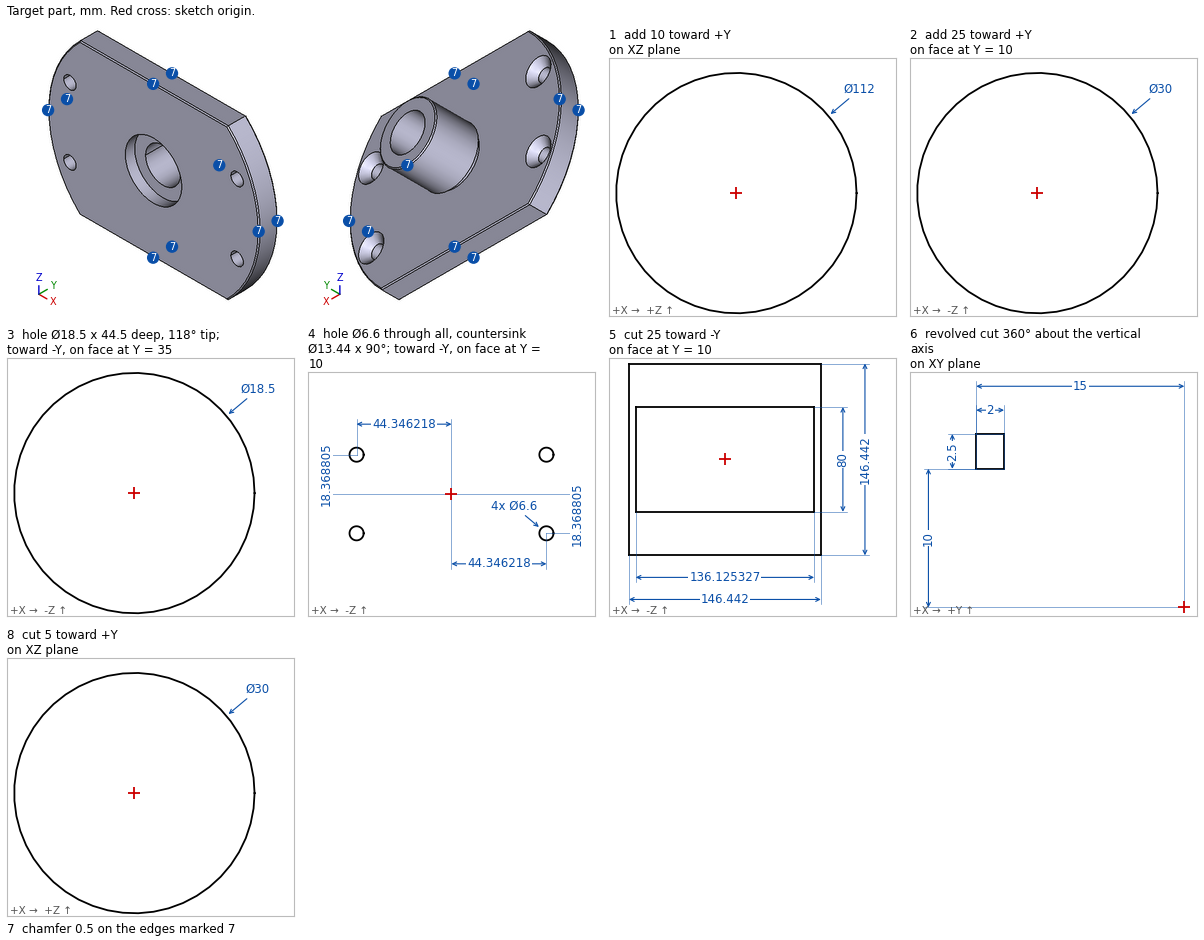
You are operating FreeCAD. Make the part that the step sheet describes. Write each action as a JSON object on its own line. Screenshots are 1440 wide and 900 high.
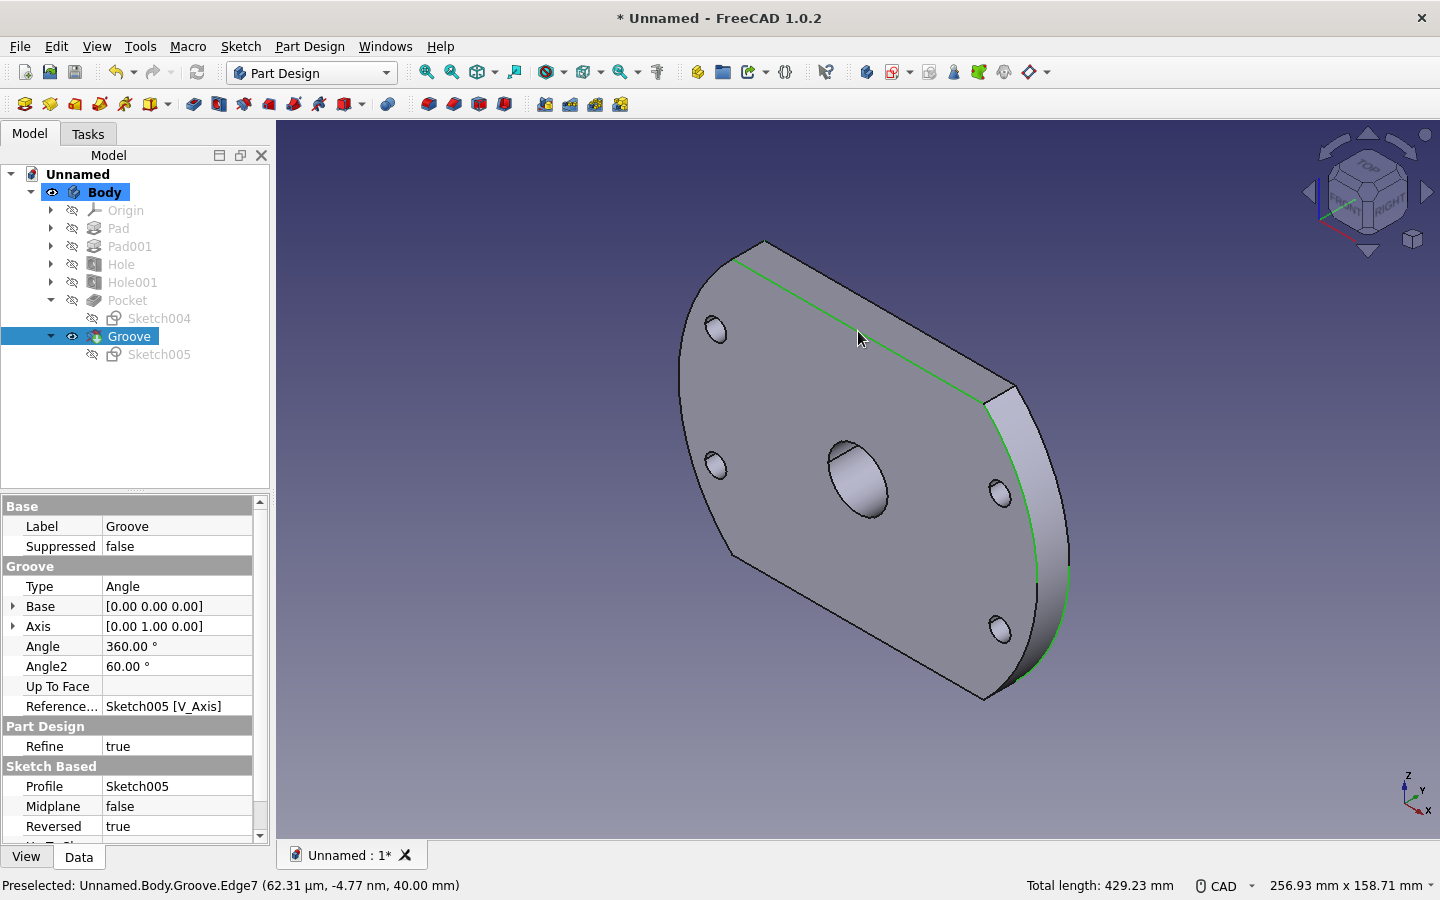
{"action": "key", "text": "2"}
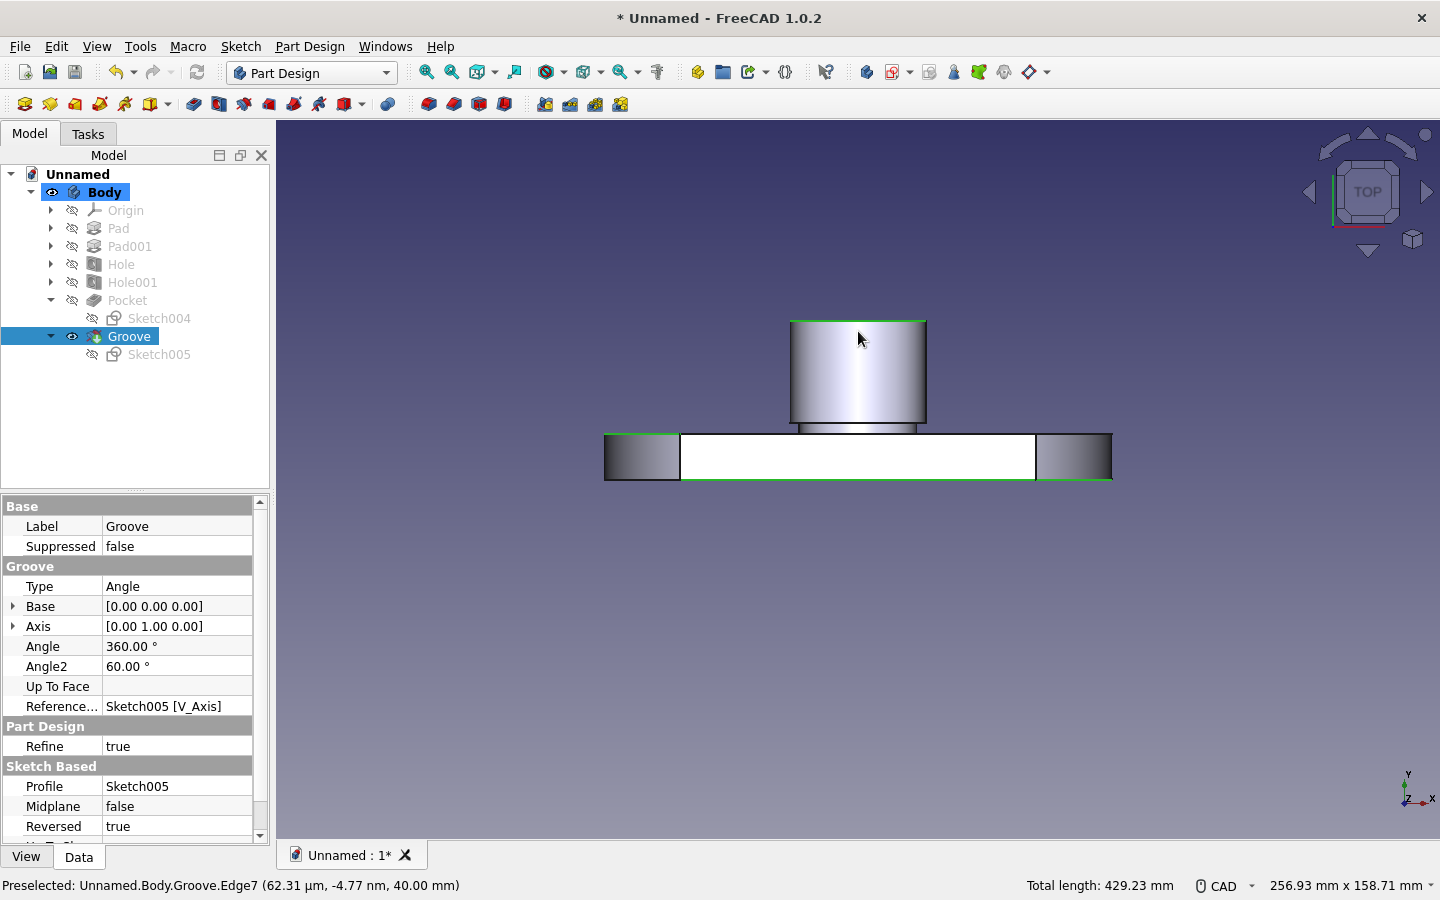
{"action": "left_click", "coordinate": [427, 72]}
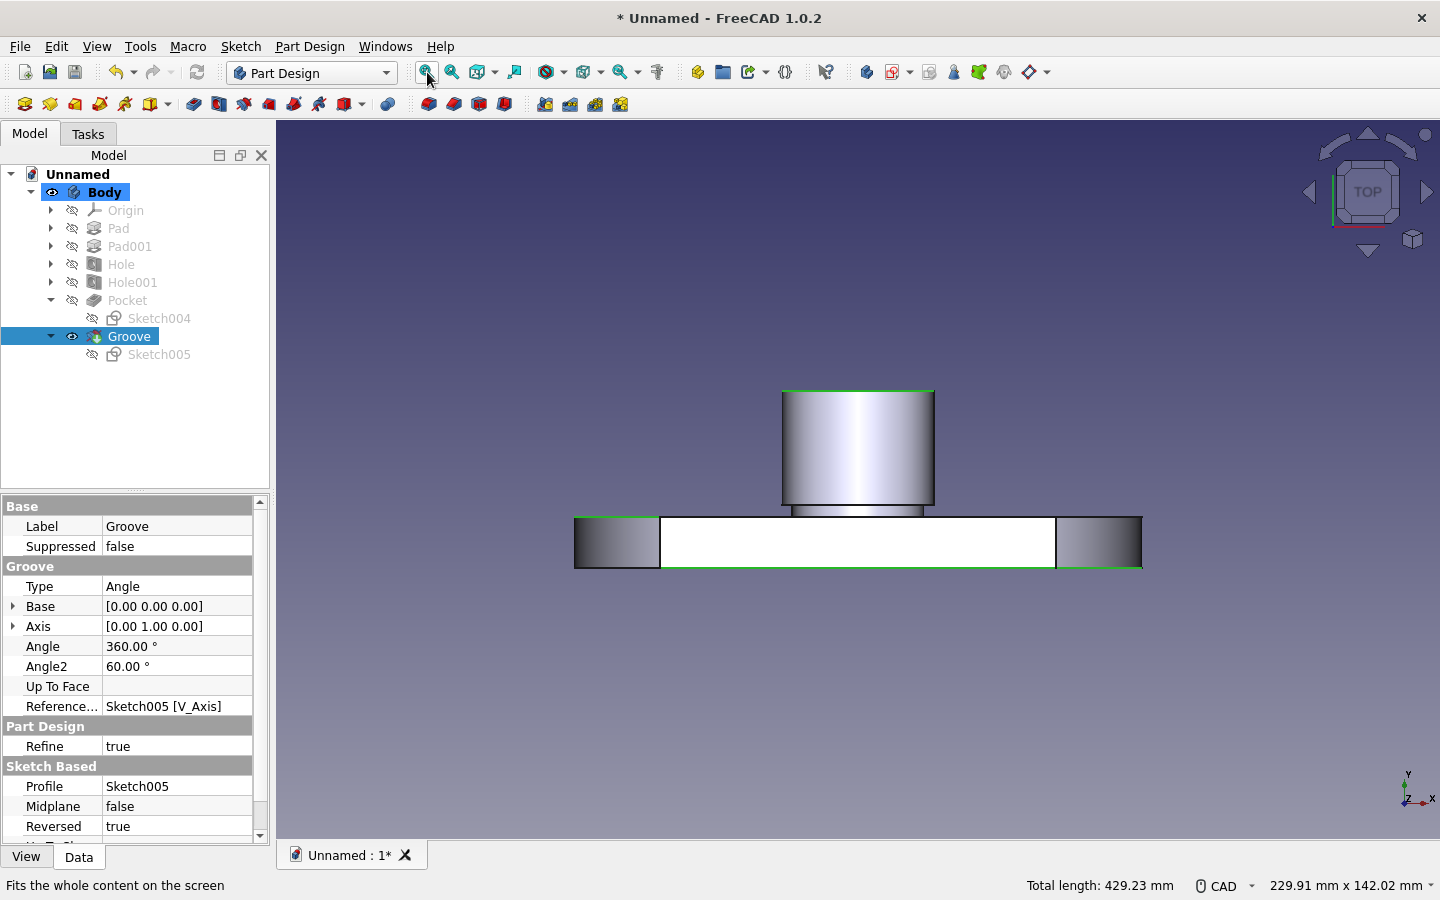
{"action": "left_click", "coordinate": [858, 516], "text": "ctrl"}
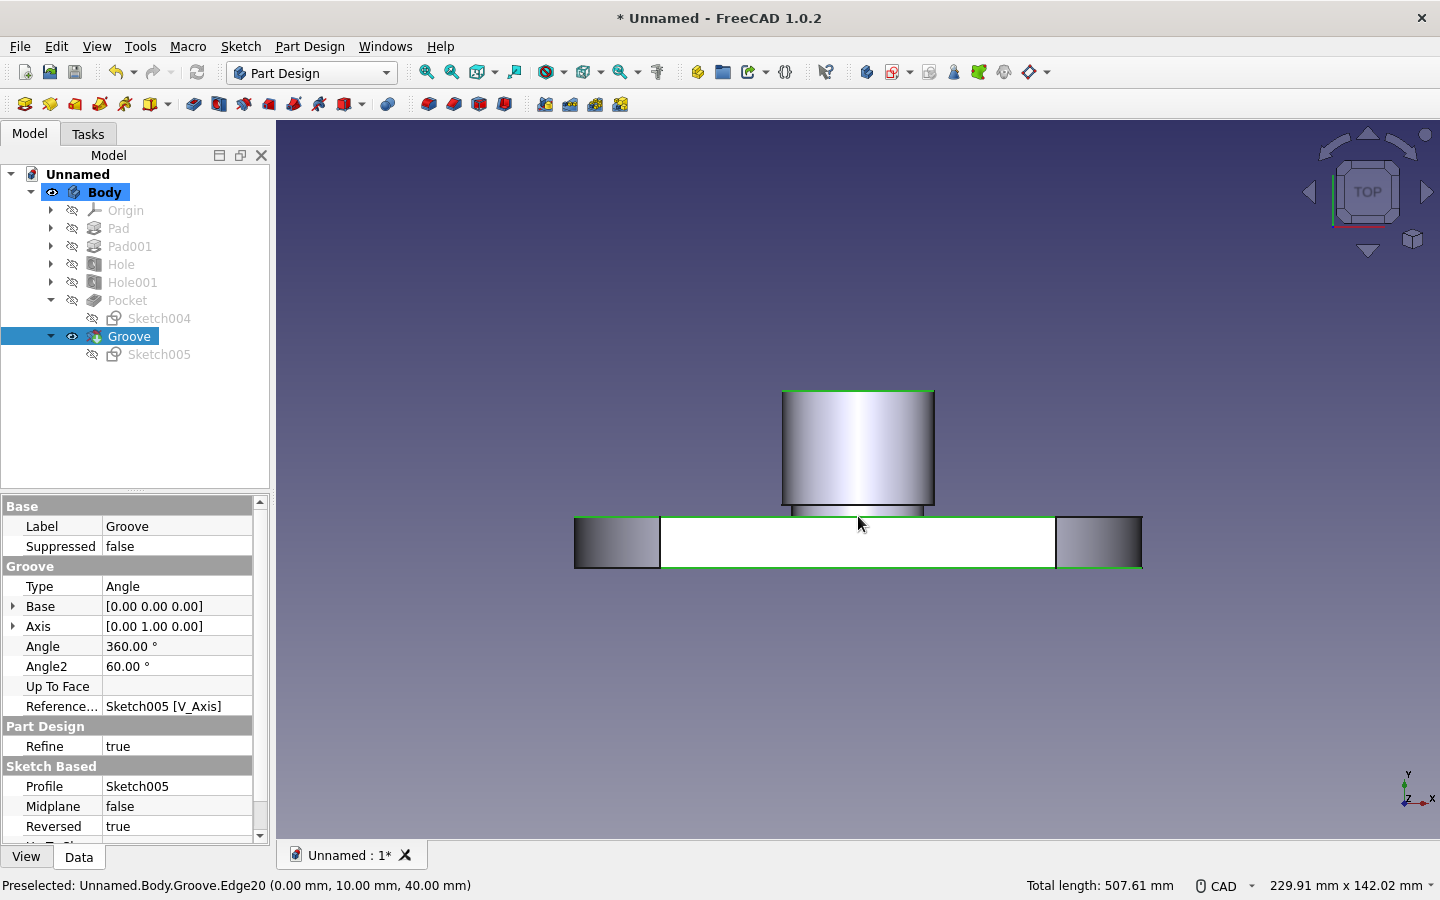
{"action": "key", "text": "1"}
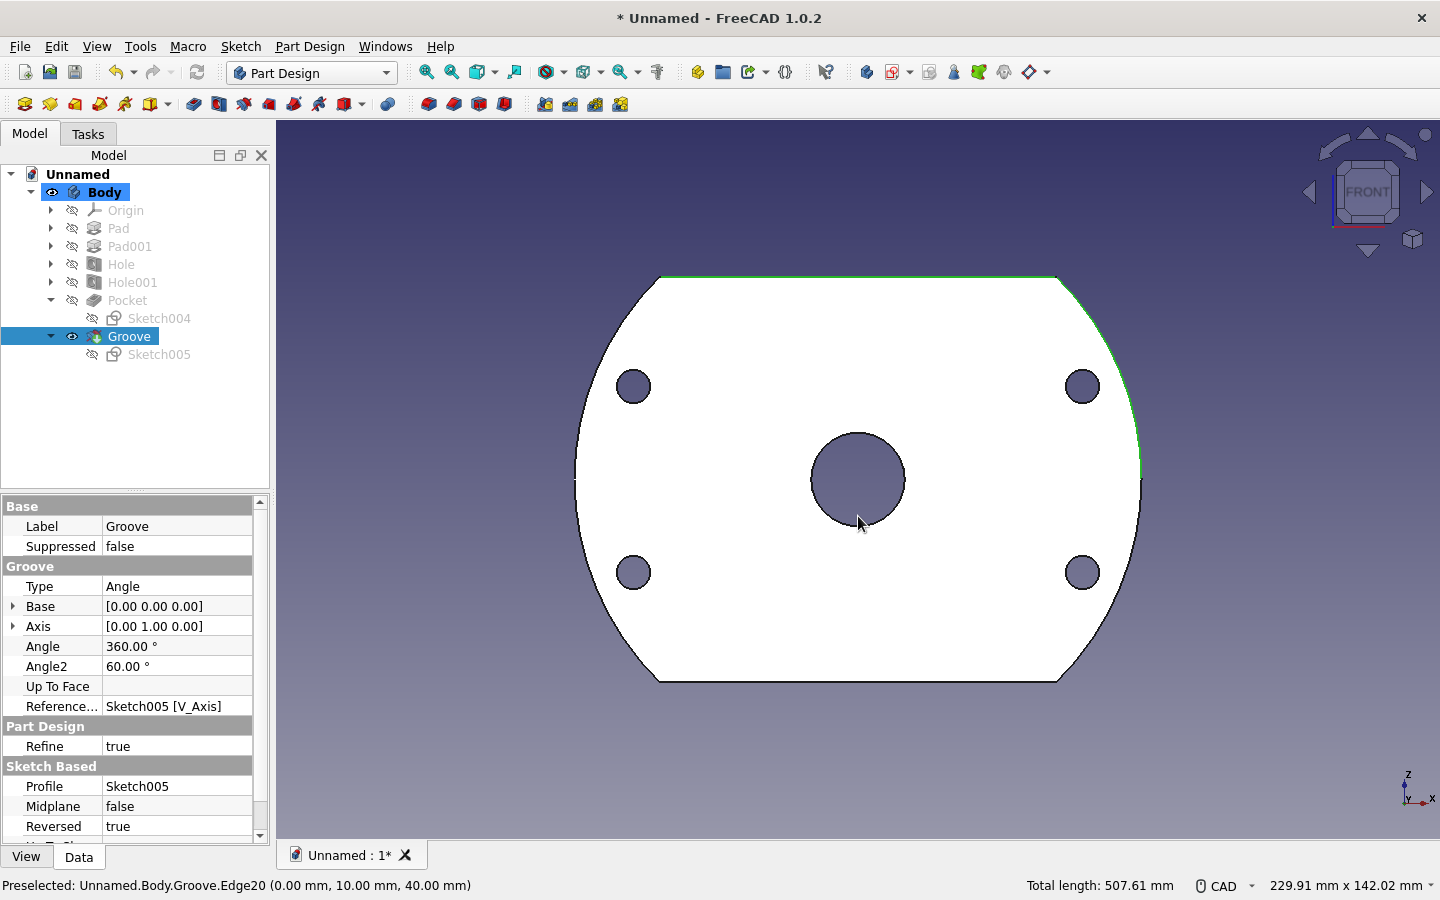
{"action": "left_click", "coordinate": [574, 478], "text": "ctrl"}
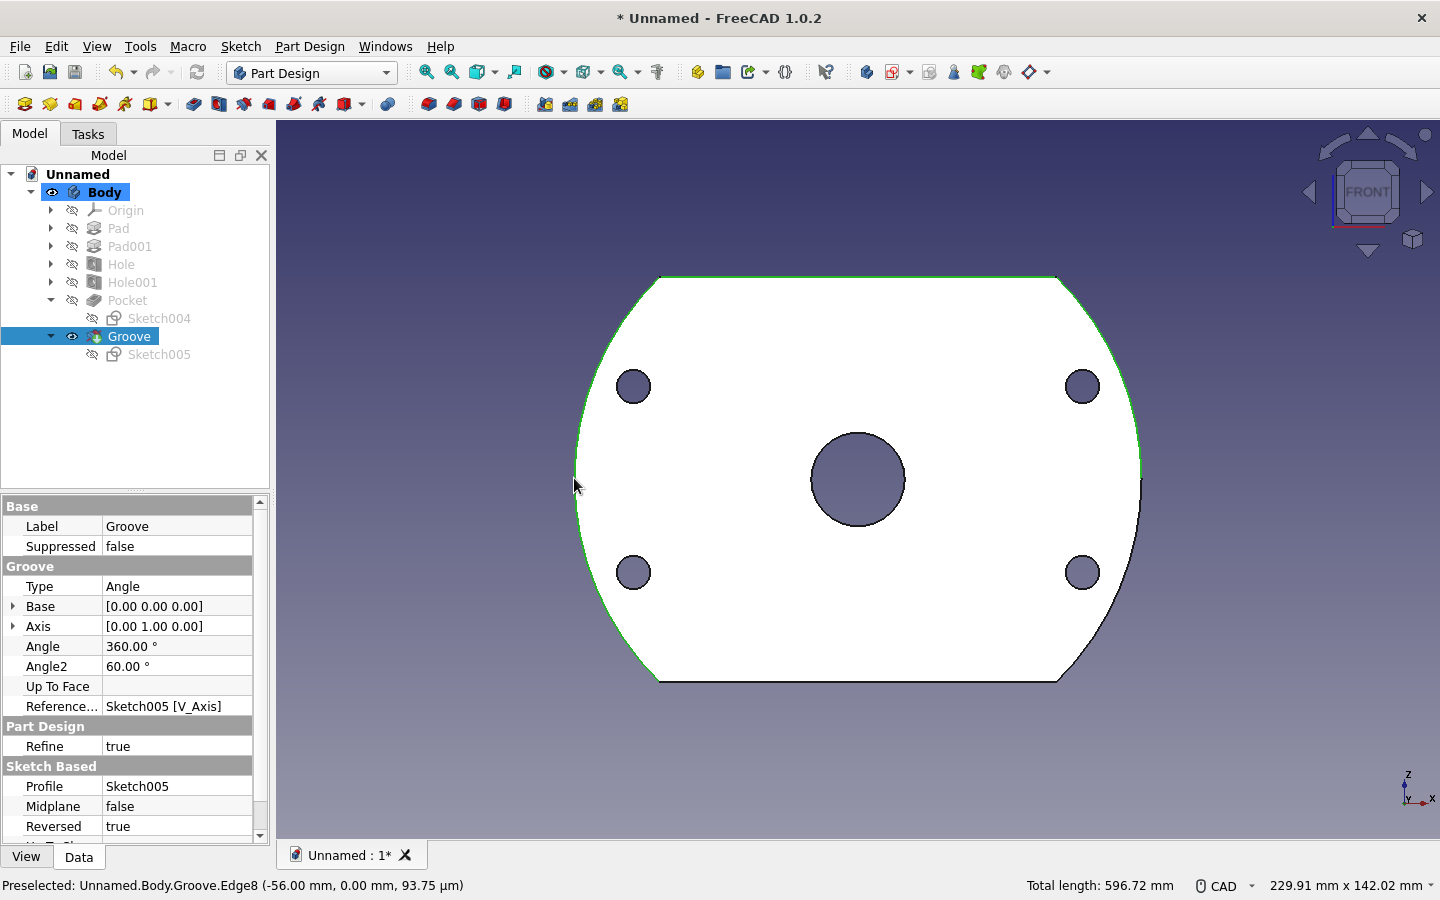
{"action": "key", "text": "3"}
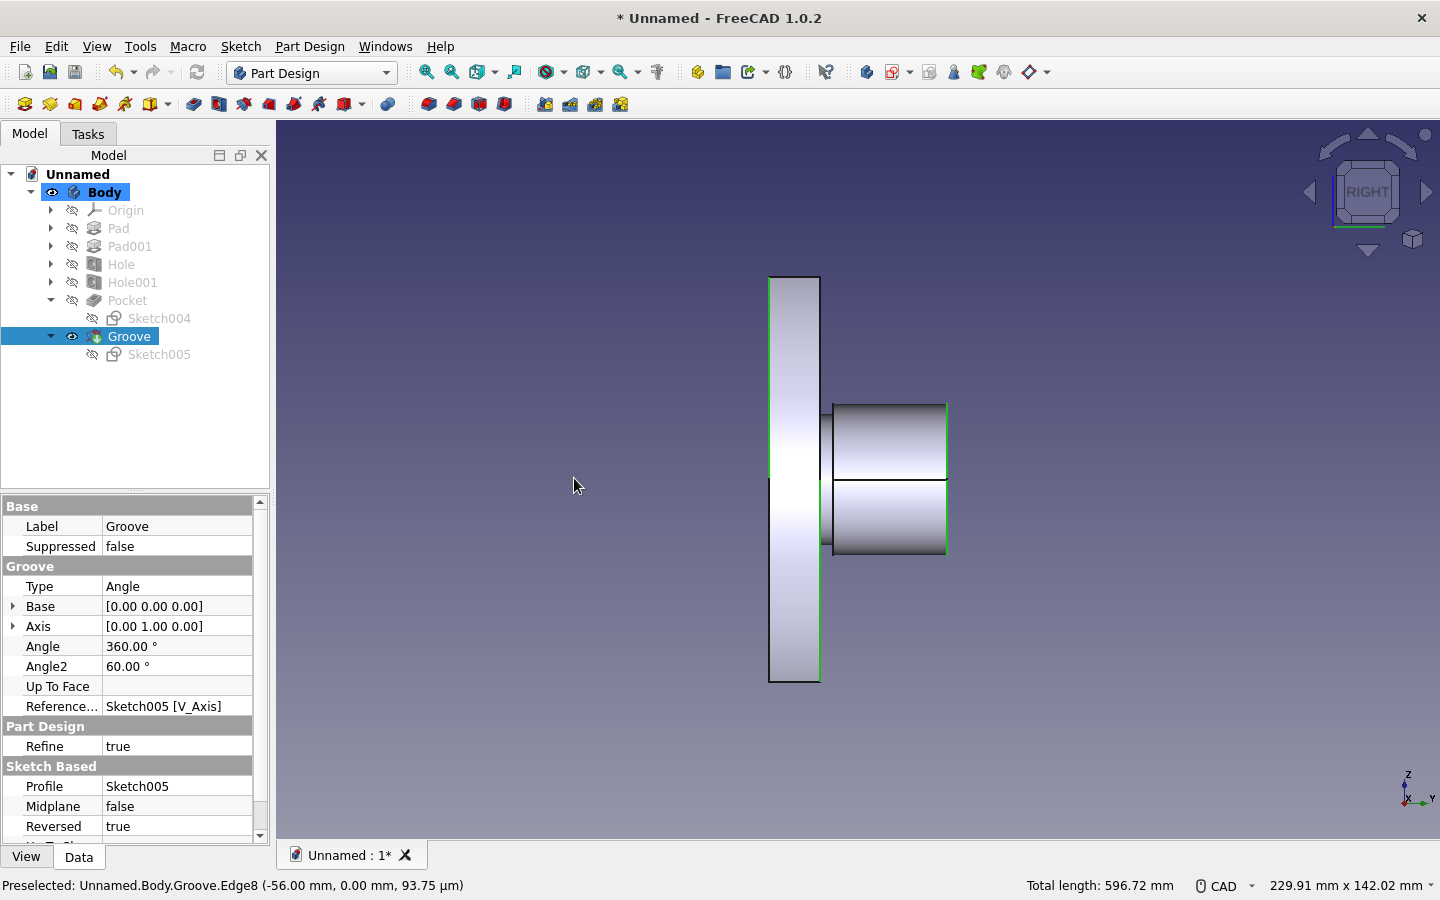
{"action": "key", "text": "5"}